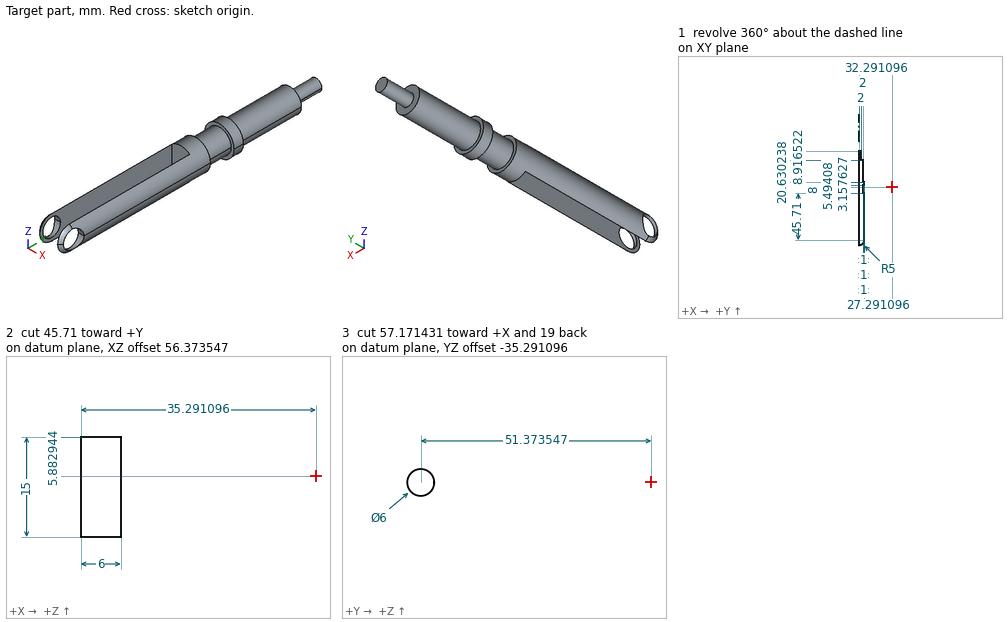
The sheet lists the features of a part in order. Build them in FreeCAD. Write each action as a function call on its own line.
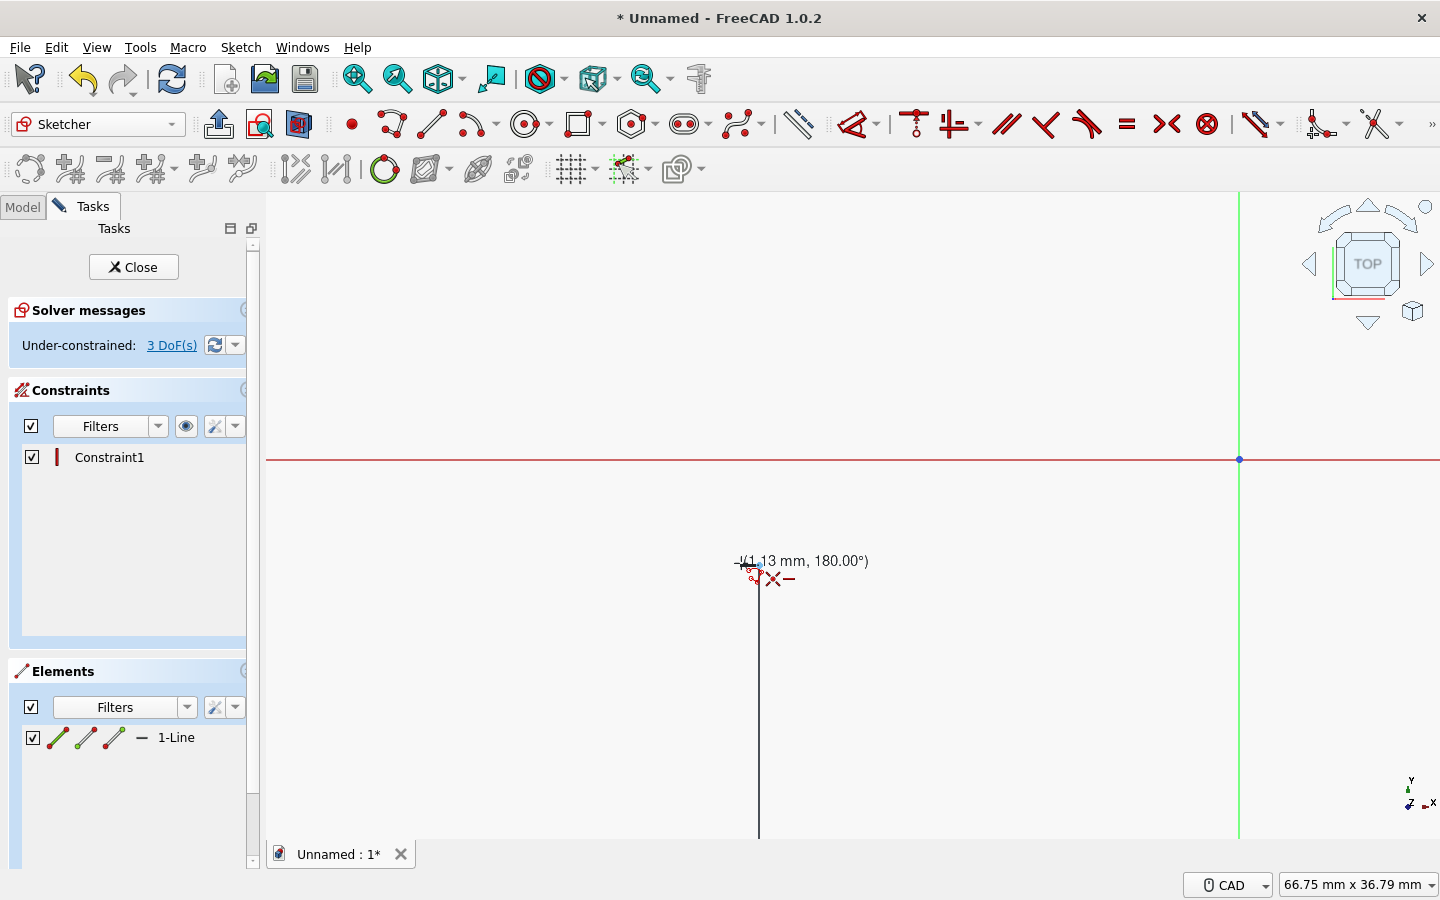
click(742, 561)
click(742, 419)
click(759, 419)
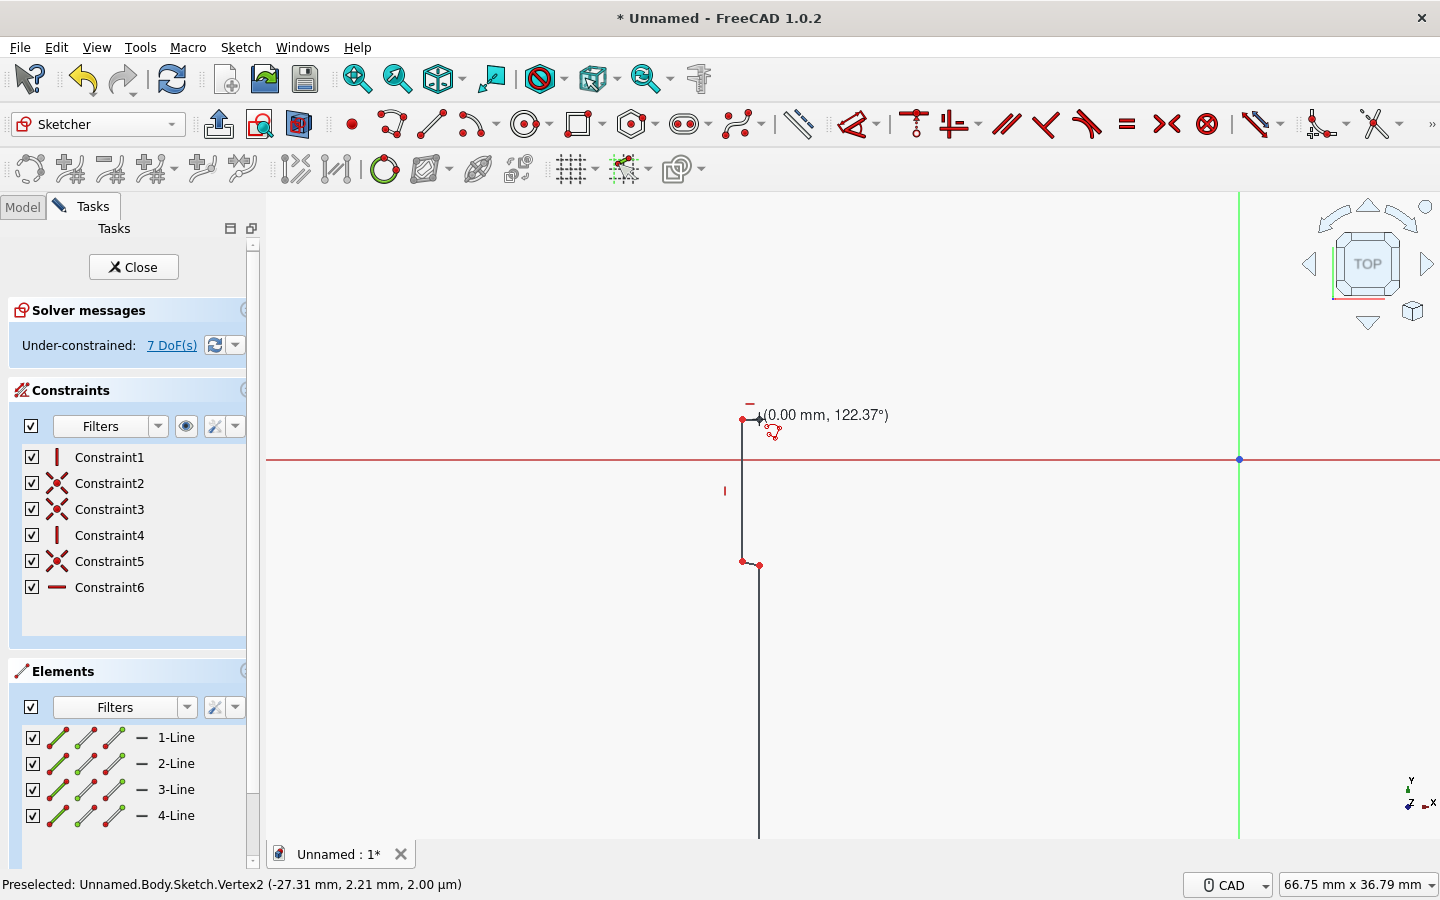
scroll(741, 563, down, 8)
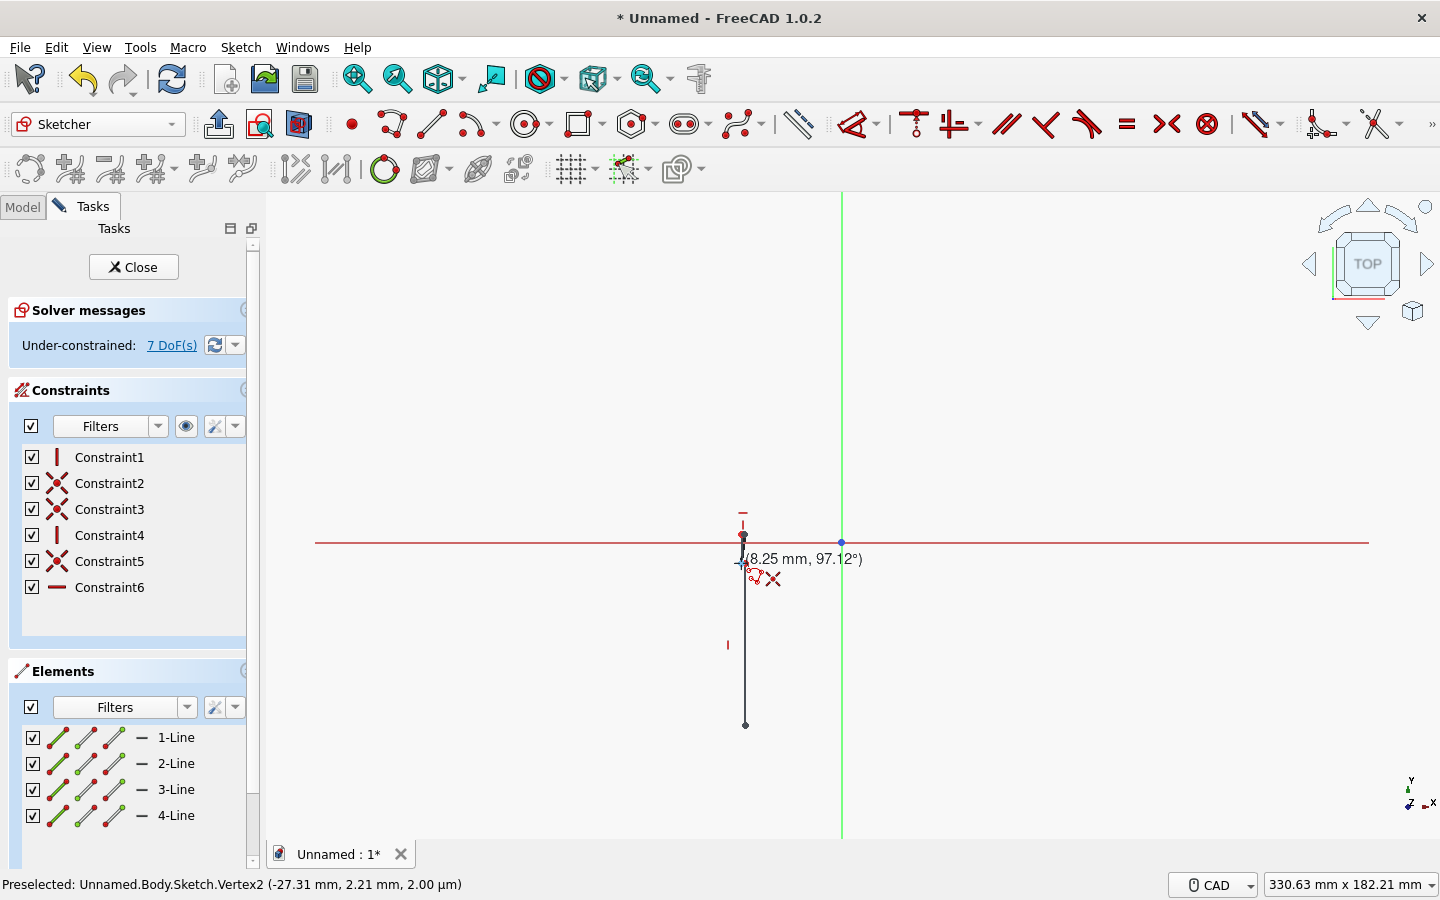
scroll(745, 523, up, 2)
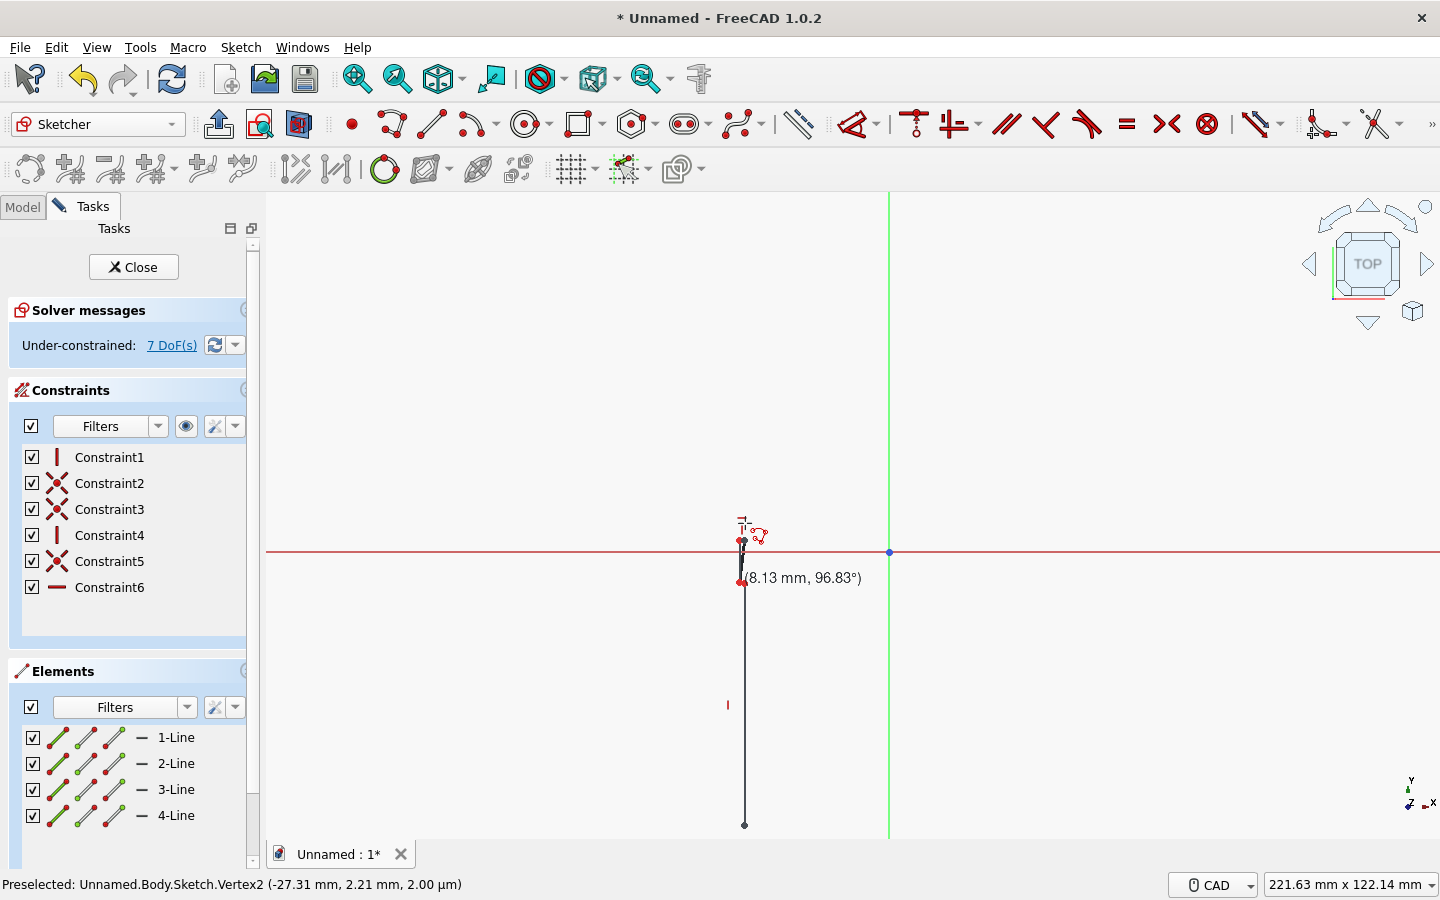
click(745, 523)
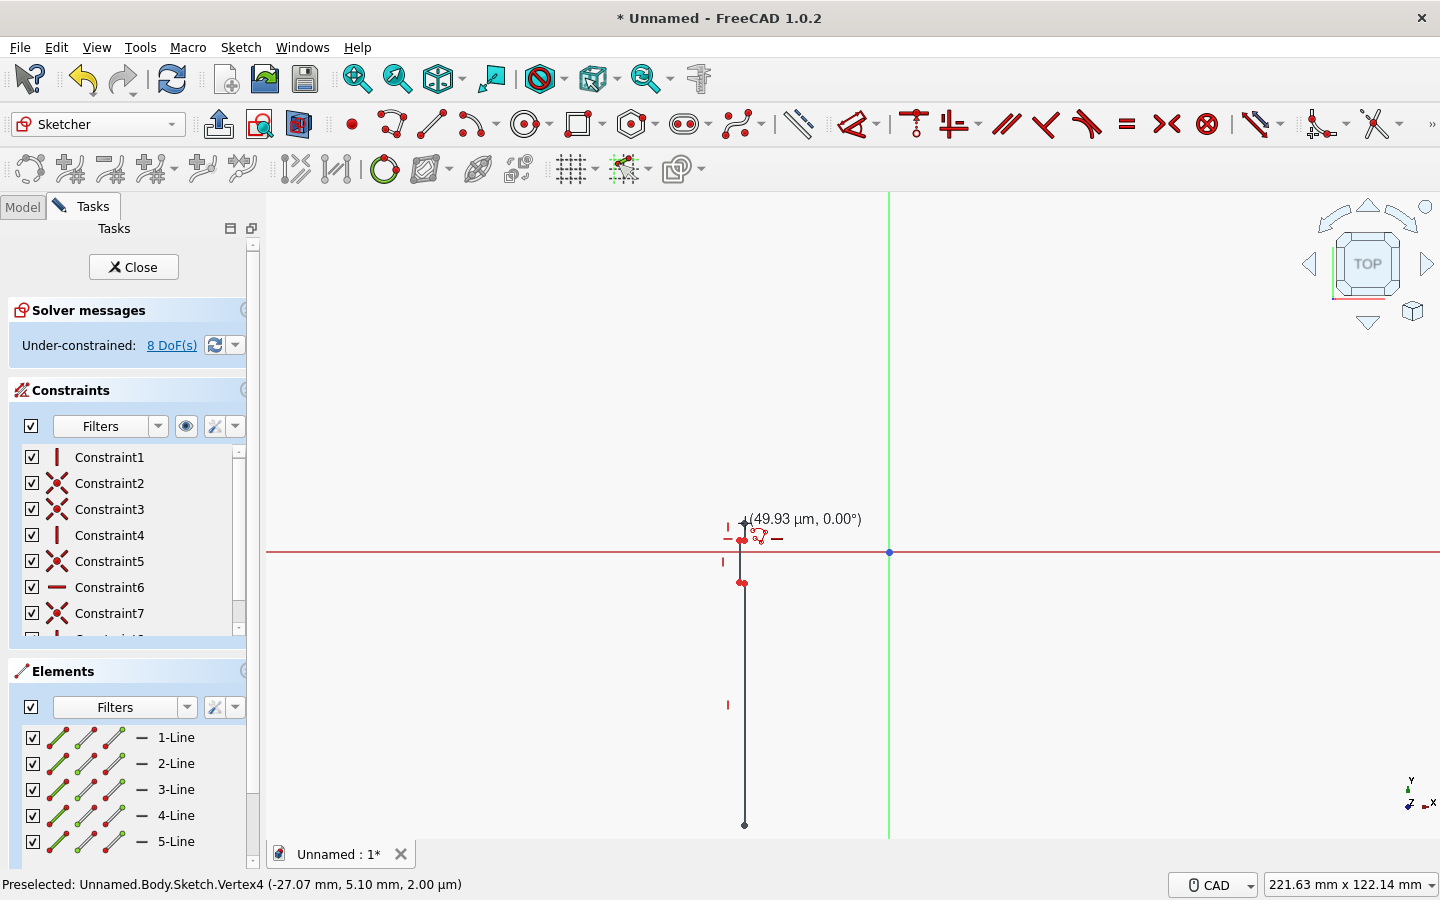
scroll(740, 523, up, 6)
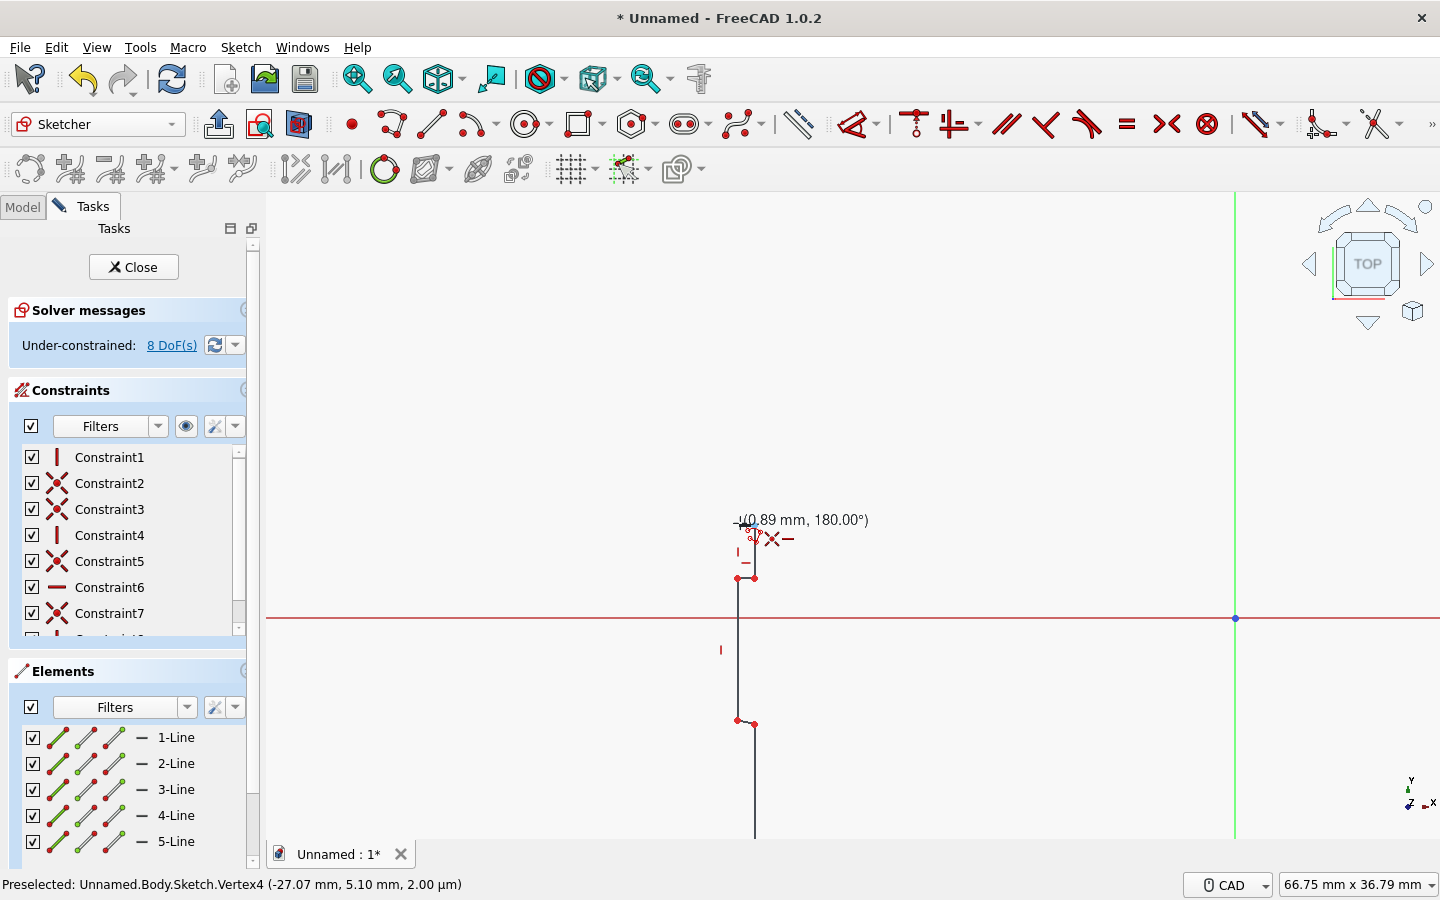
click(738, 522)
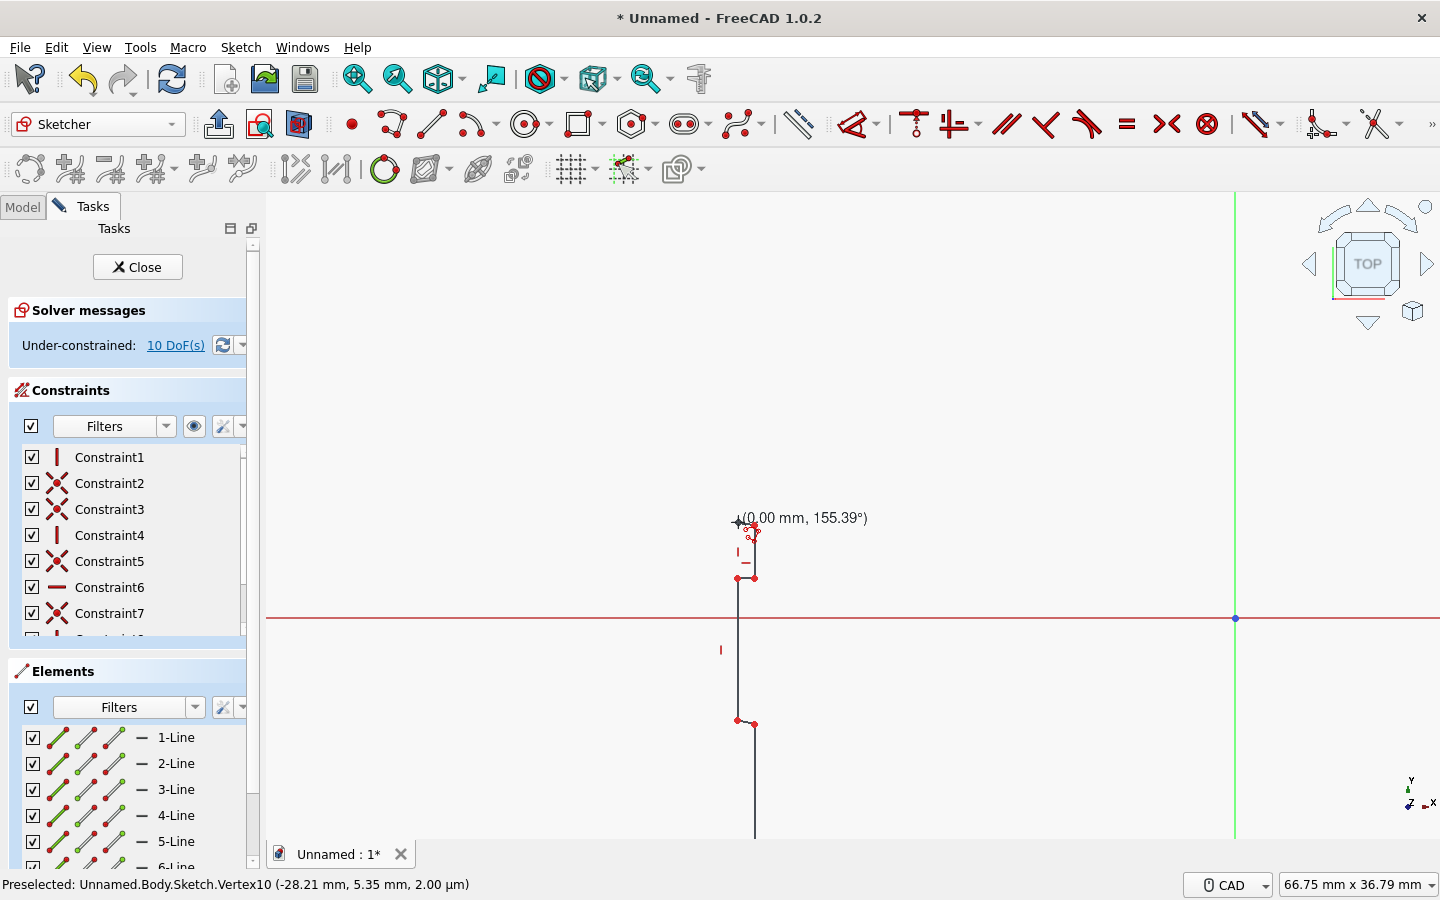
scroll(742, 523, down, 8)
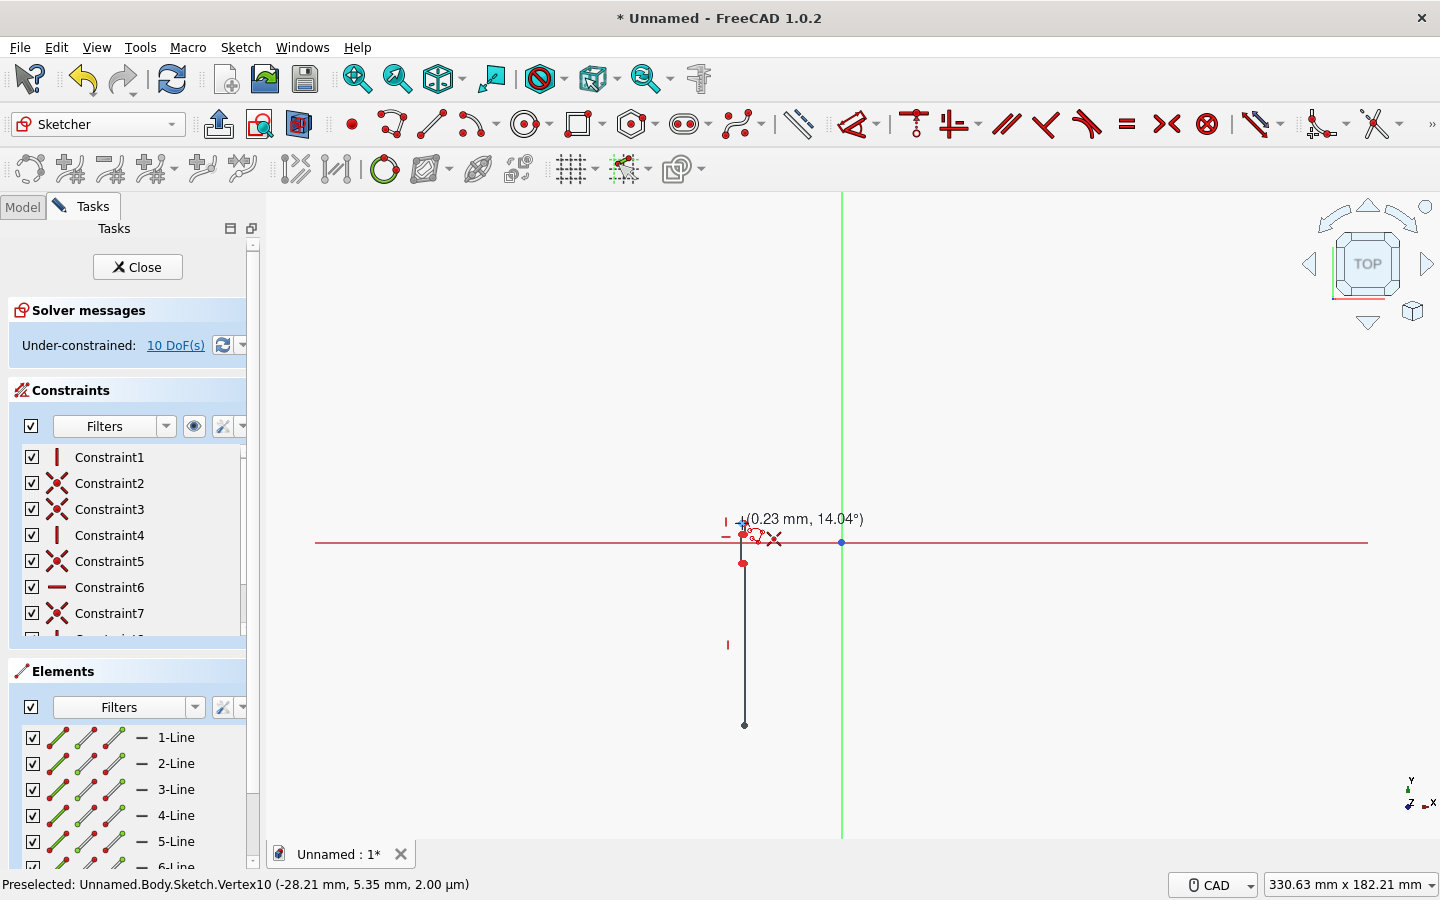
click(742, 450)